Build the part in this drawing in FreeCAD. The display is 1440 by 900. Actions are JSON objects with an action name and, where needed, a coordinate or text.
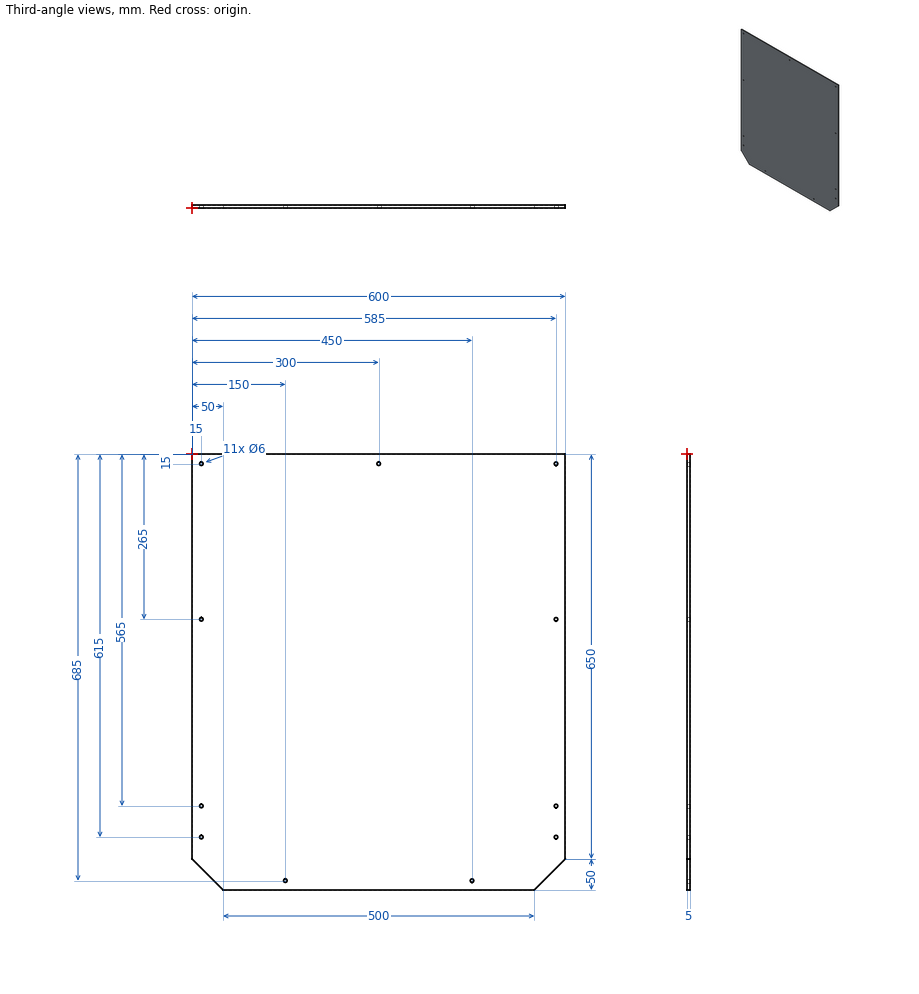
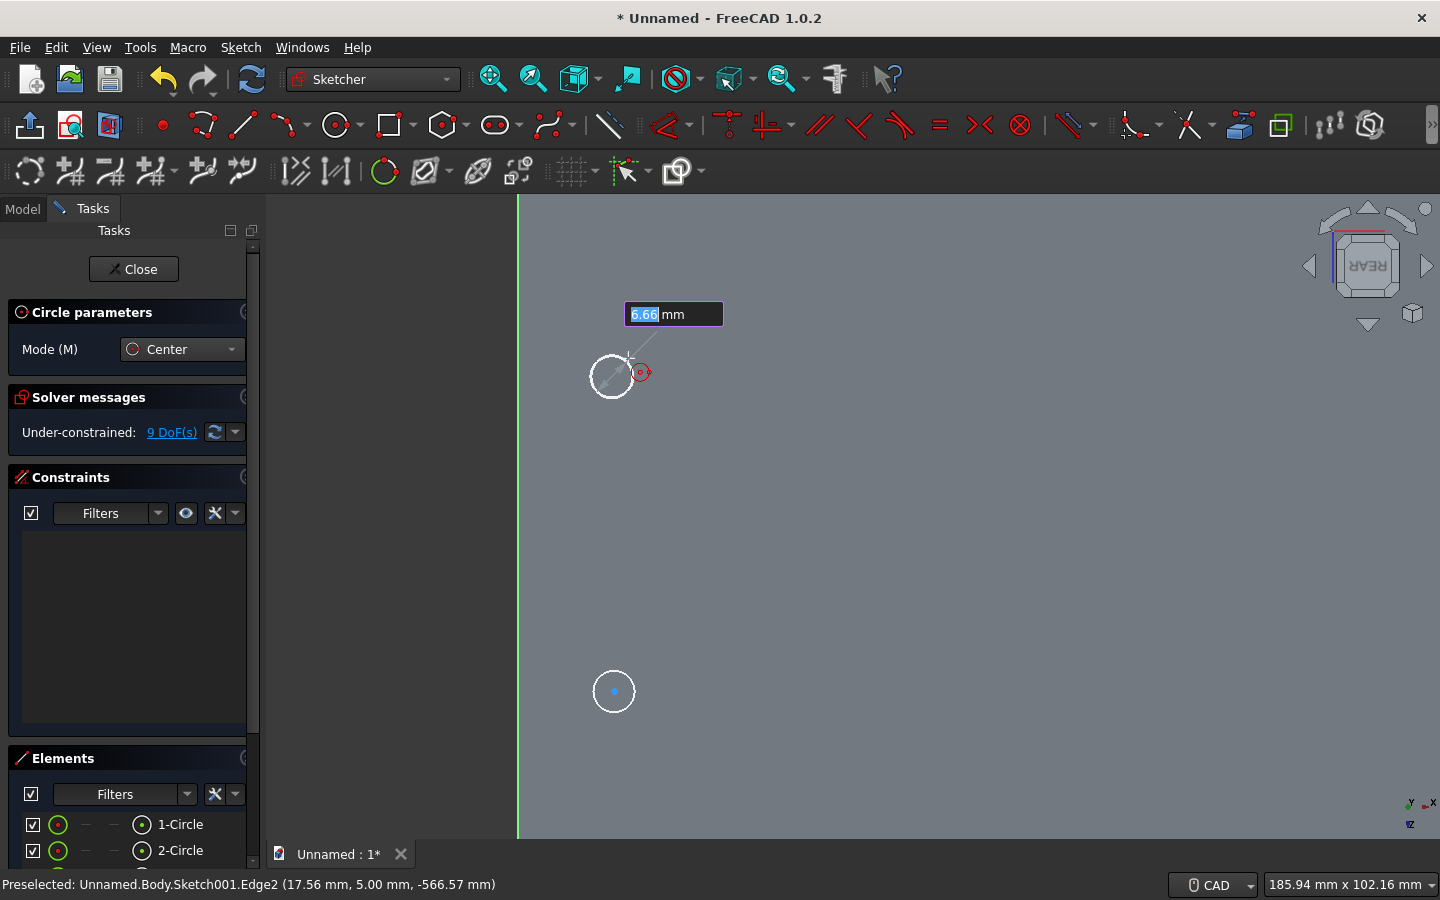
{"action": "left_click", "coordinate": [626, 358]}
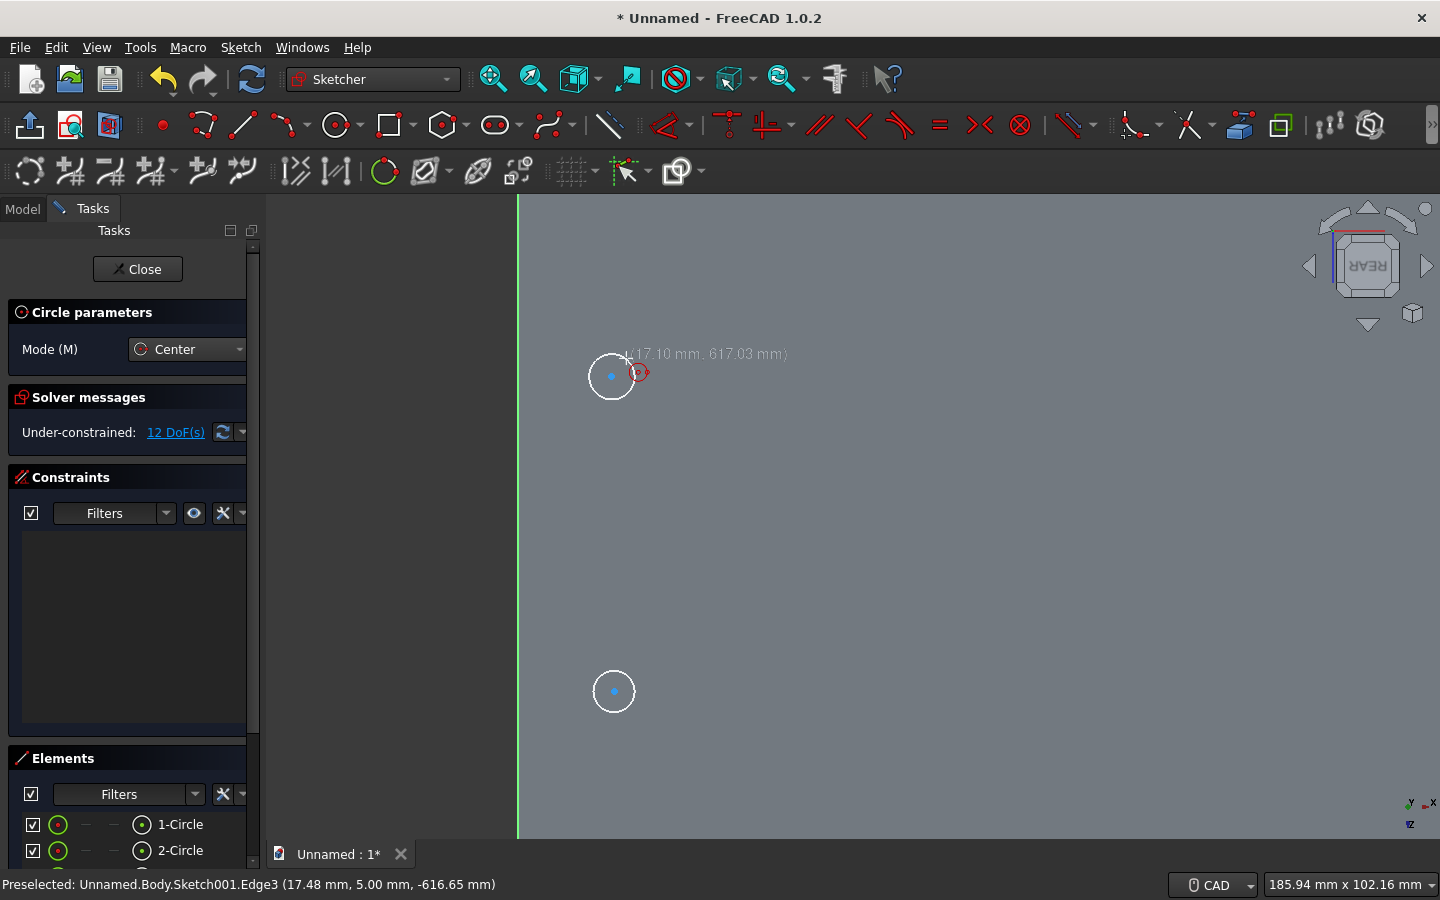
{"action": "scroll", "coordinate": [626, 360], "scroll_direction": "down", "scroll_amount": 12}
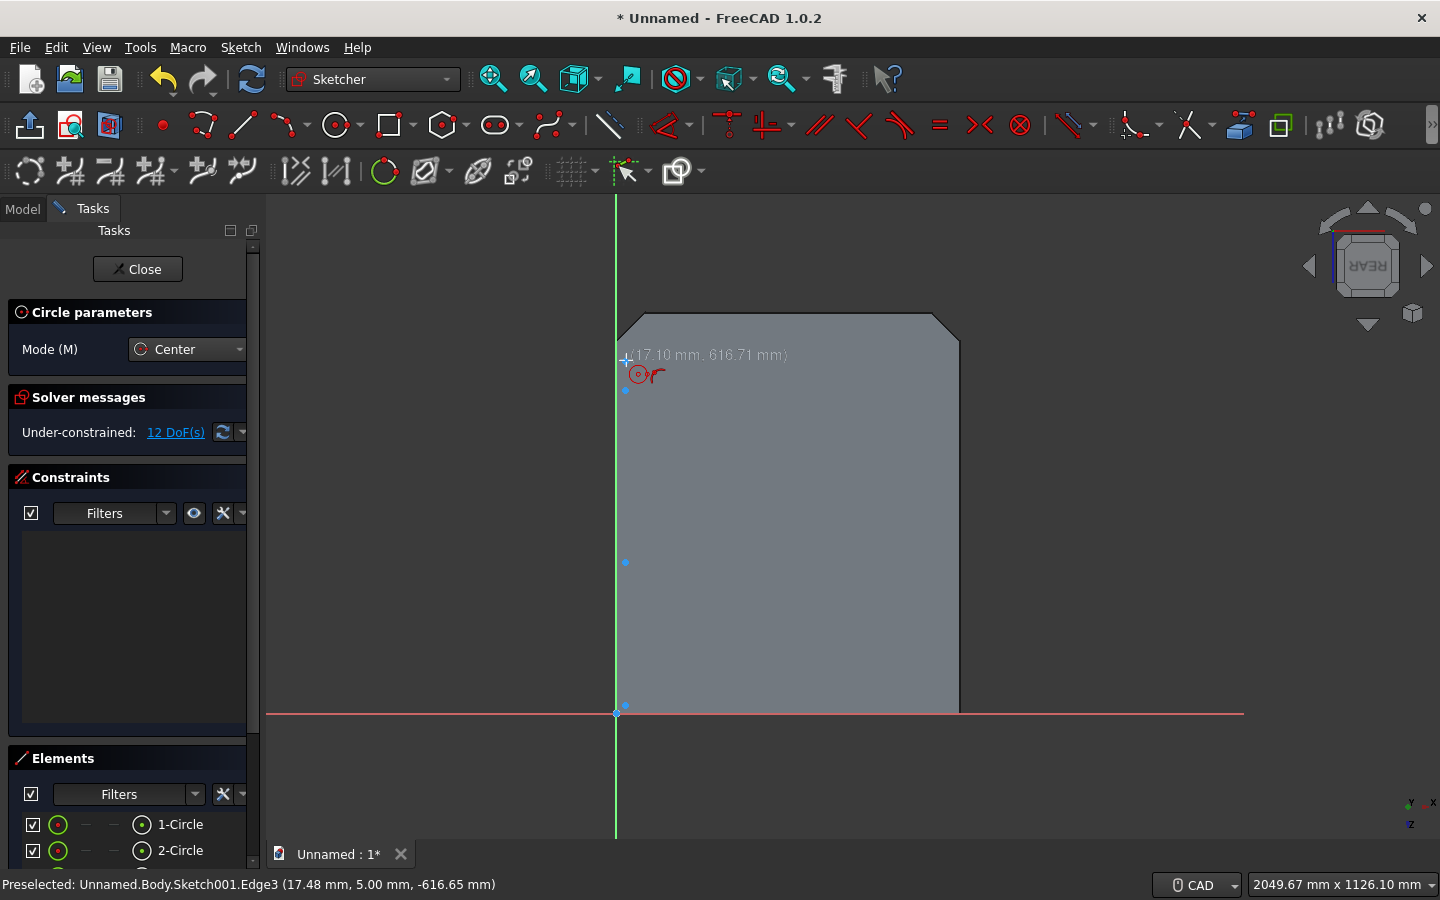
{"action": "scroll", "coordinate": [702, 321], "scroll_direction": "up", "scroll_amount": 13}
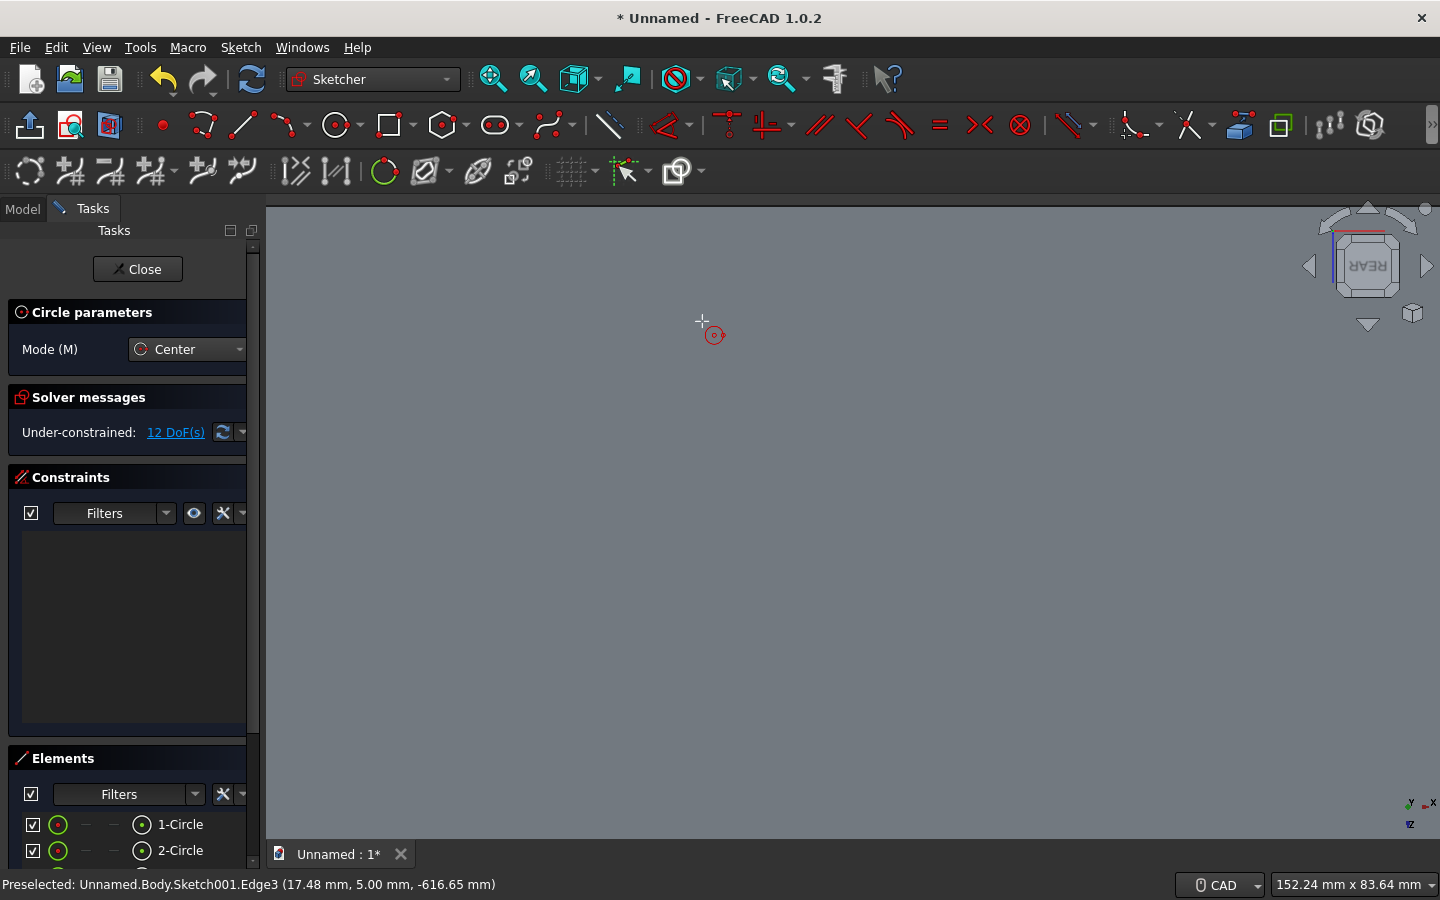
{"action": "scroll", "coordinate": [702, 321], "scroll_direction": "down", "scroll_amount": 13}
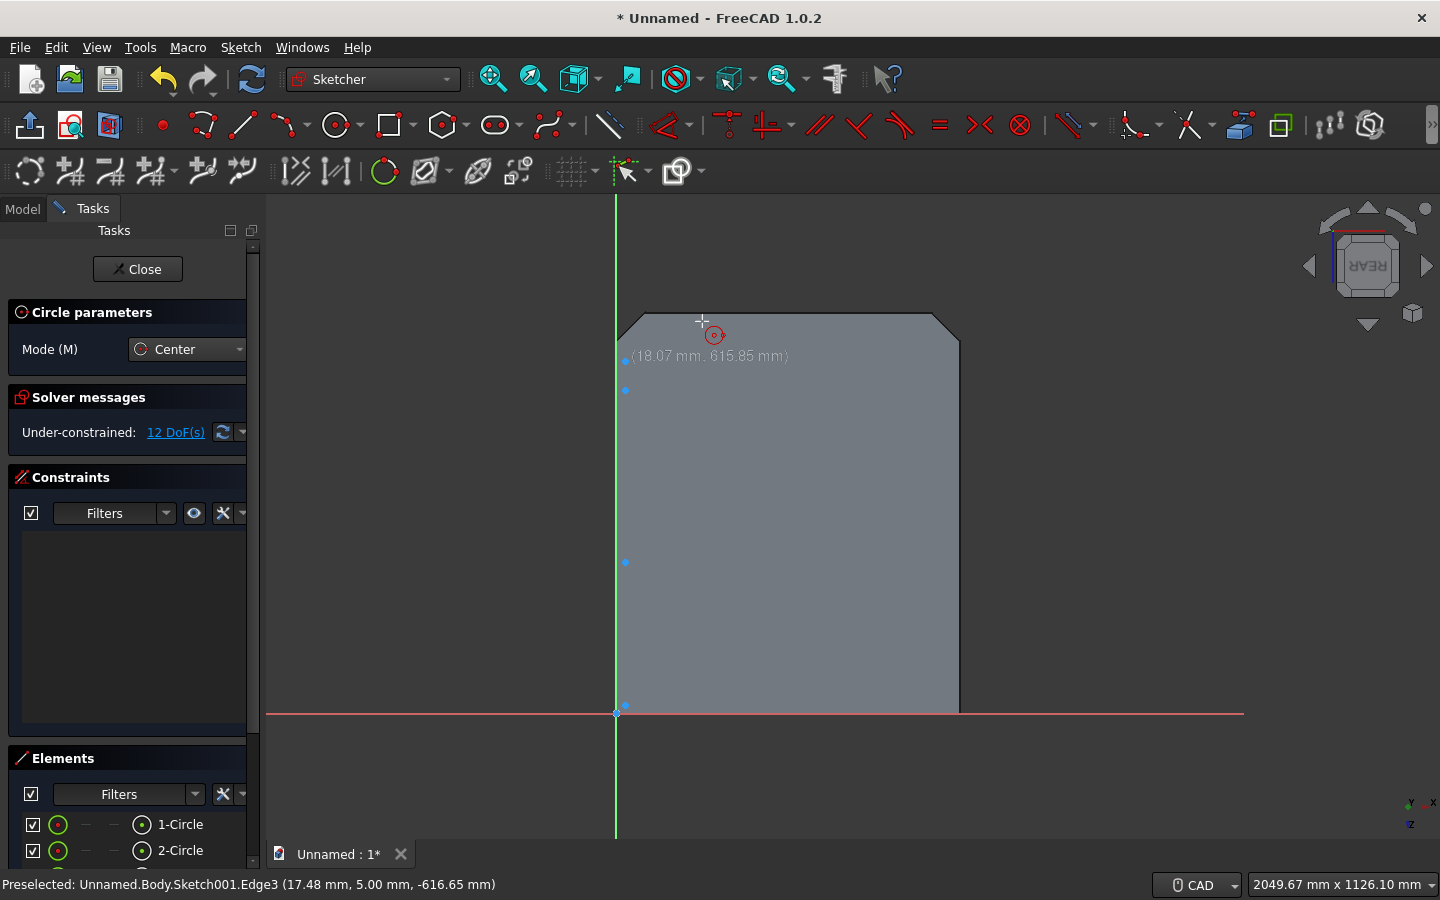
{"action": "left_click", "coordinate": [702, 321]}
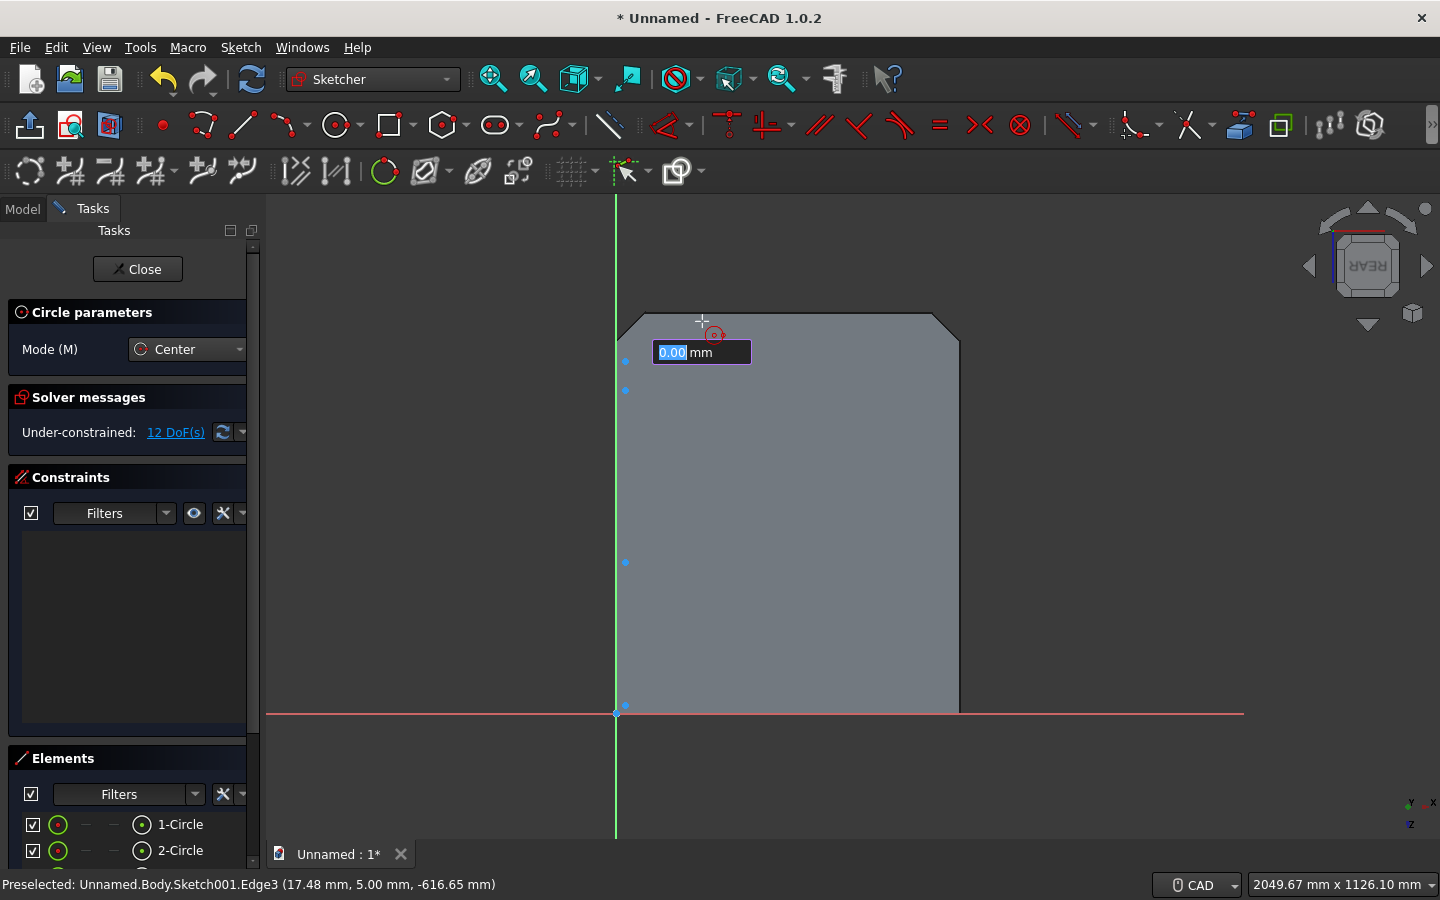
{"action": "scroll", "coordinate": [704, 320], "scroll_direction": "up", "scroll_amount": 12}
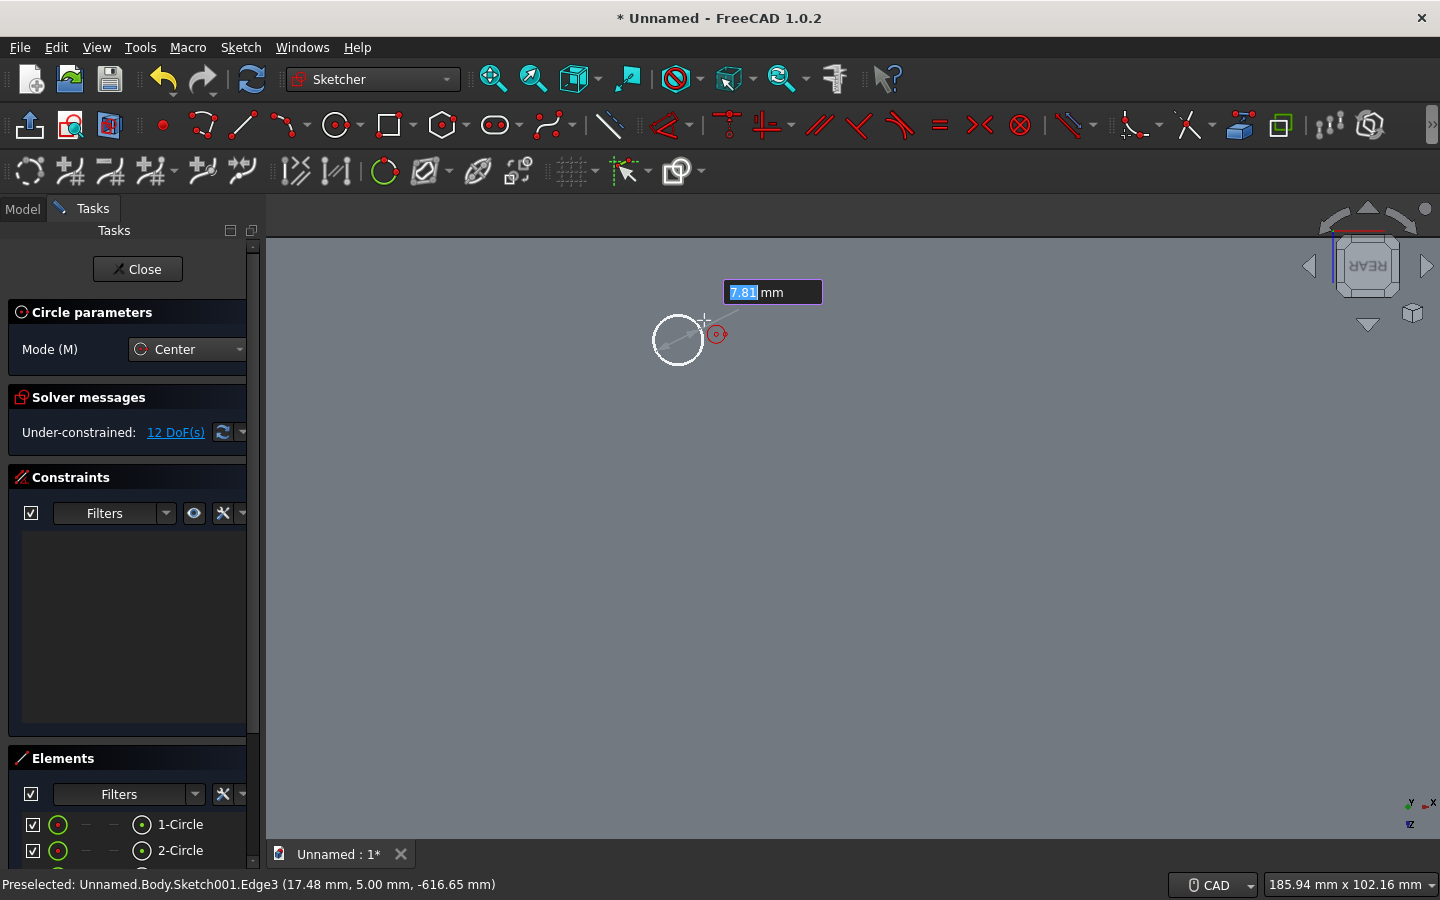
{"action": "left_click", "coordinate": [696, 318]}